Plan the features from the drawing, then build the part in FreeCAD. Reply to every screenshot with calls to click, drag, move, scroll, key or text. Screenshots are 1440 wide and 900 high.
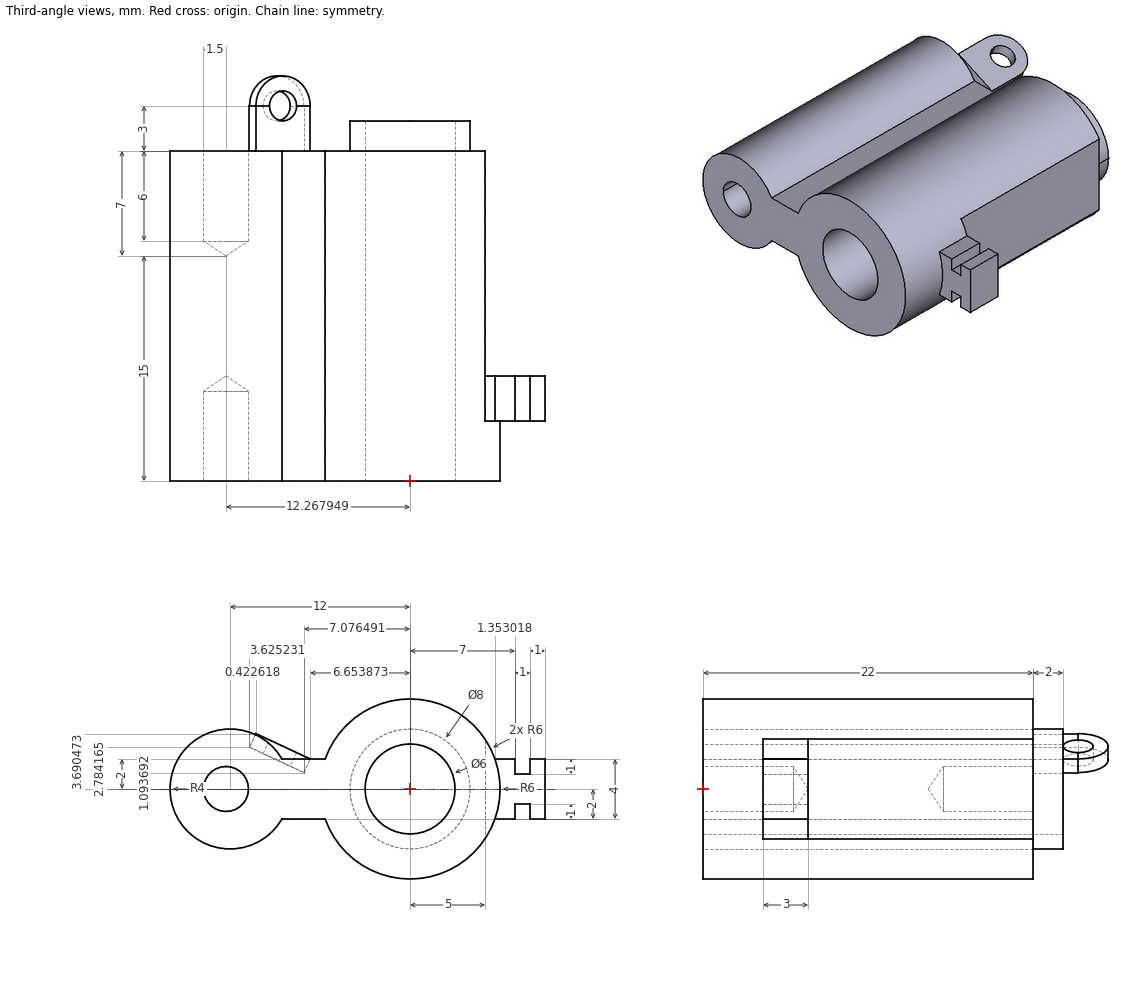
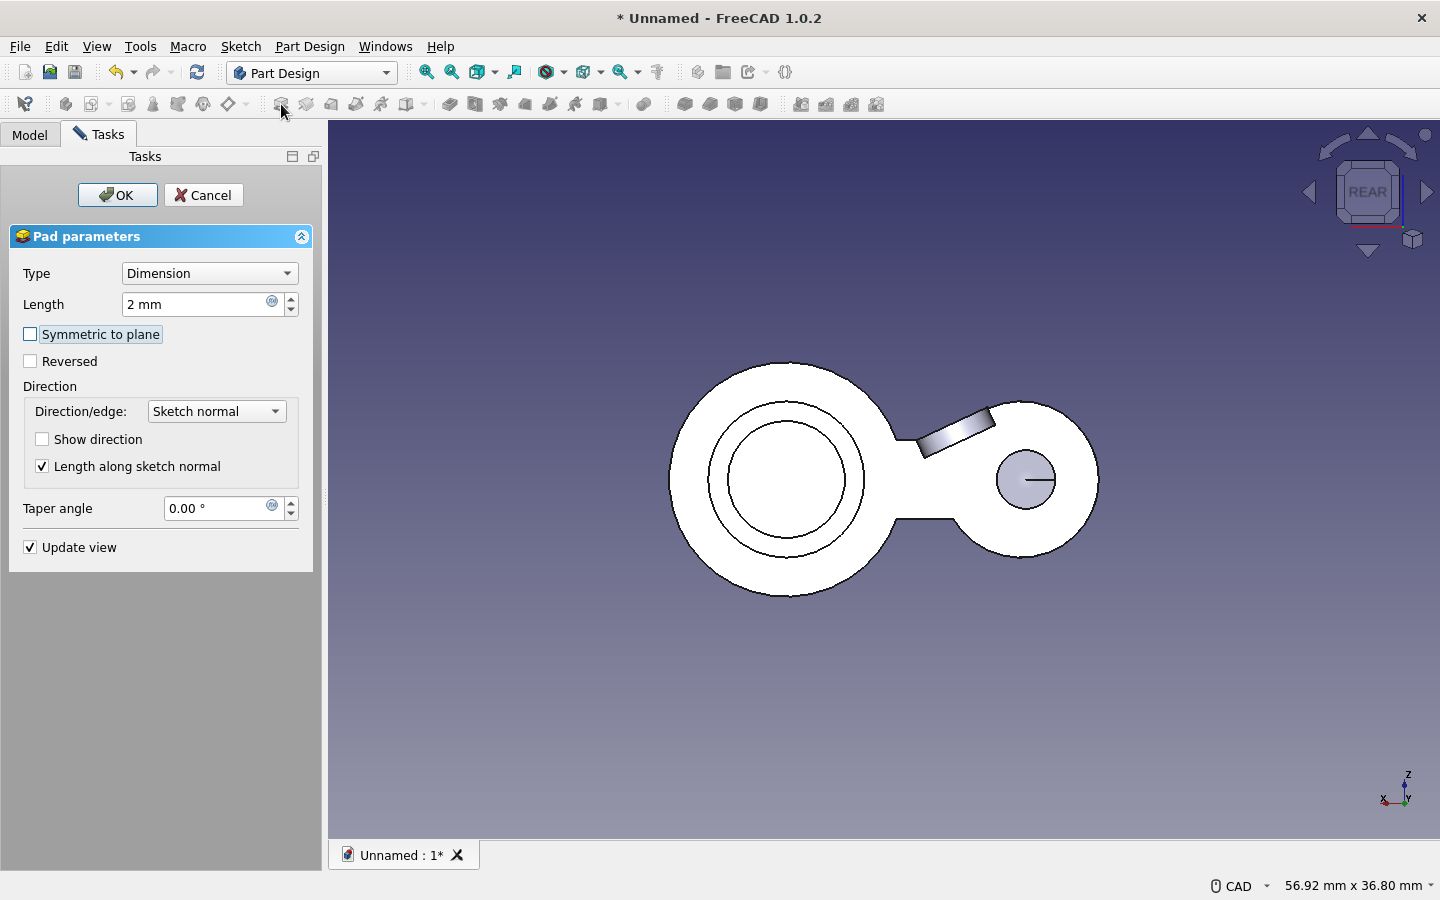
click(118, 195)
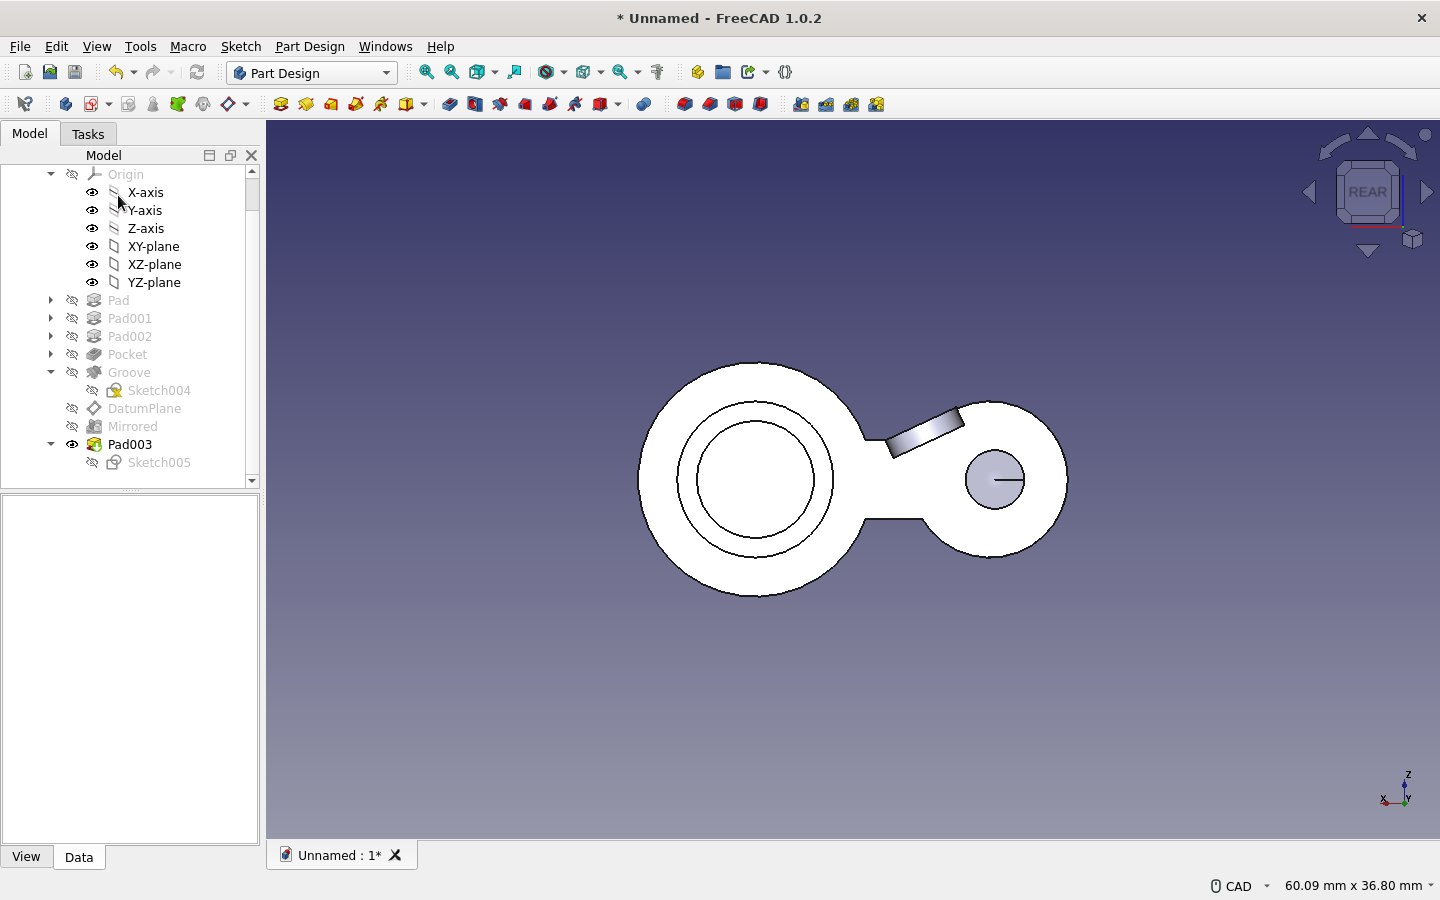
click(427, 72)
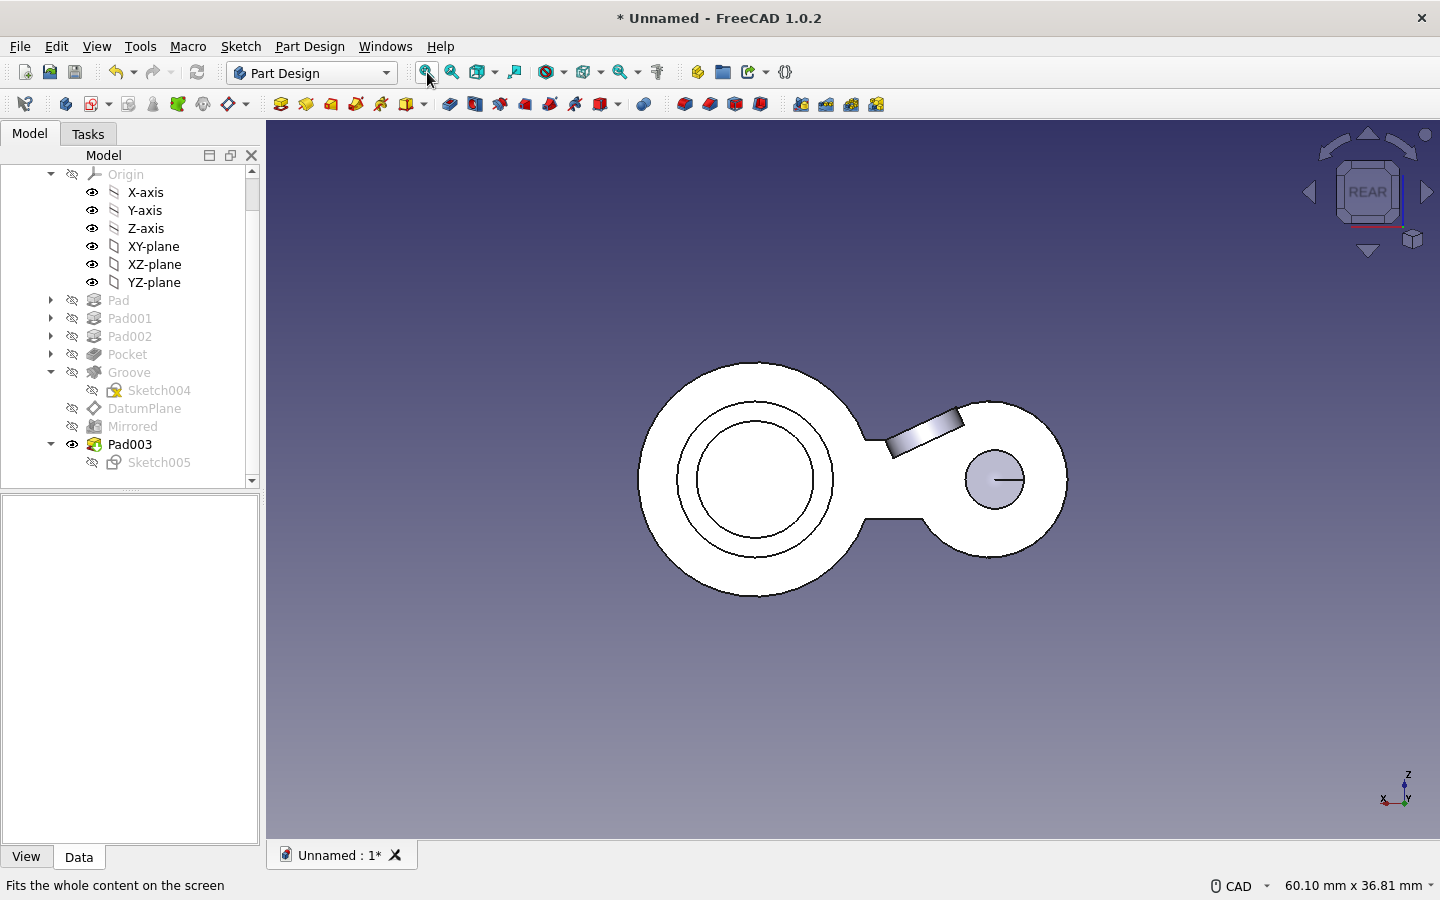
click(914, 478)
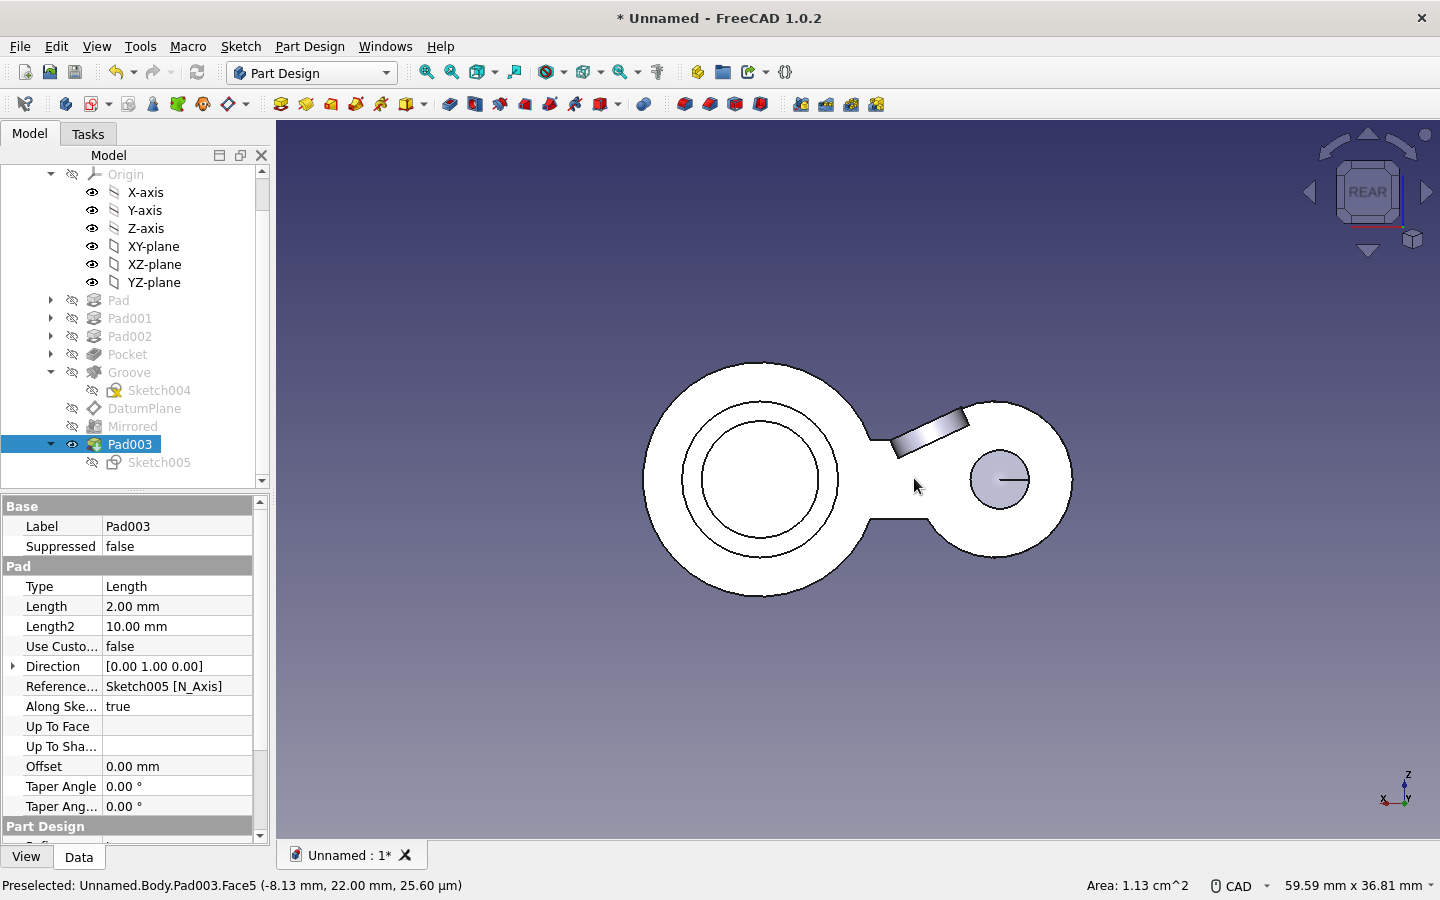
click(90, 104)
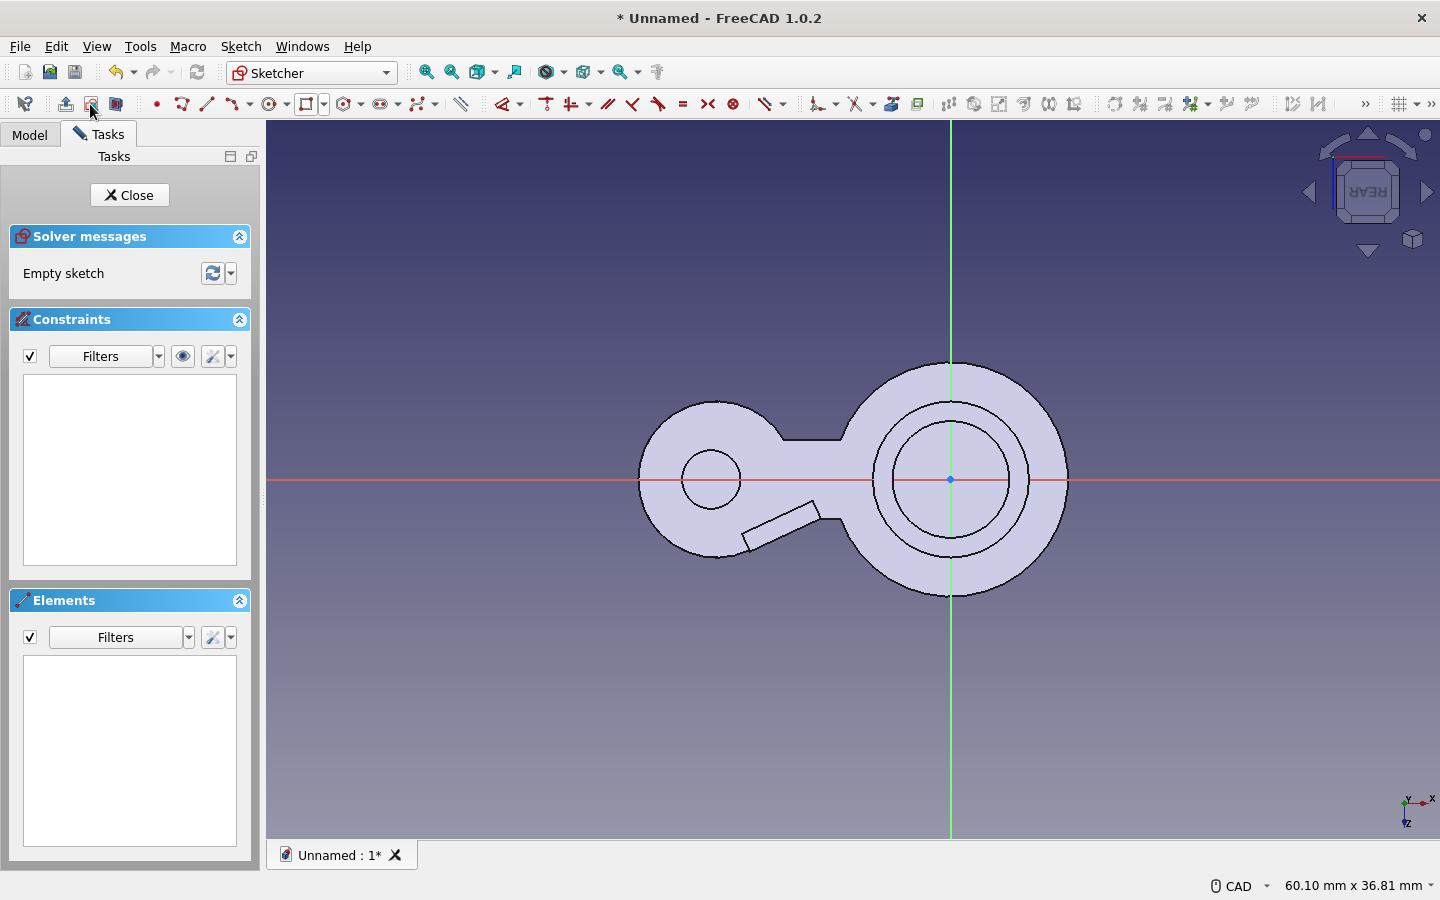
click(116, 104)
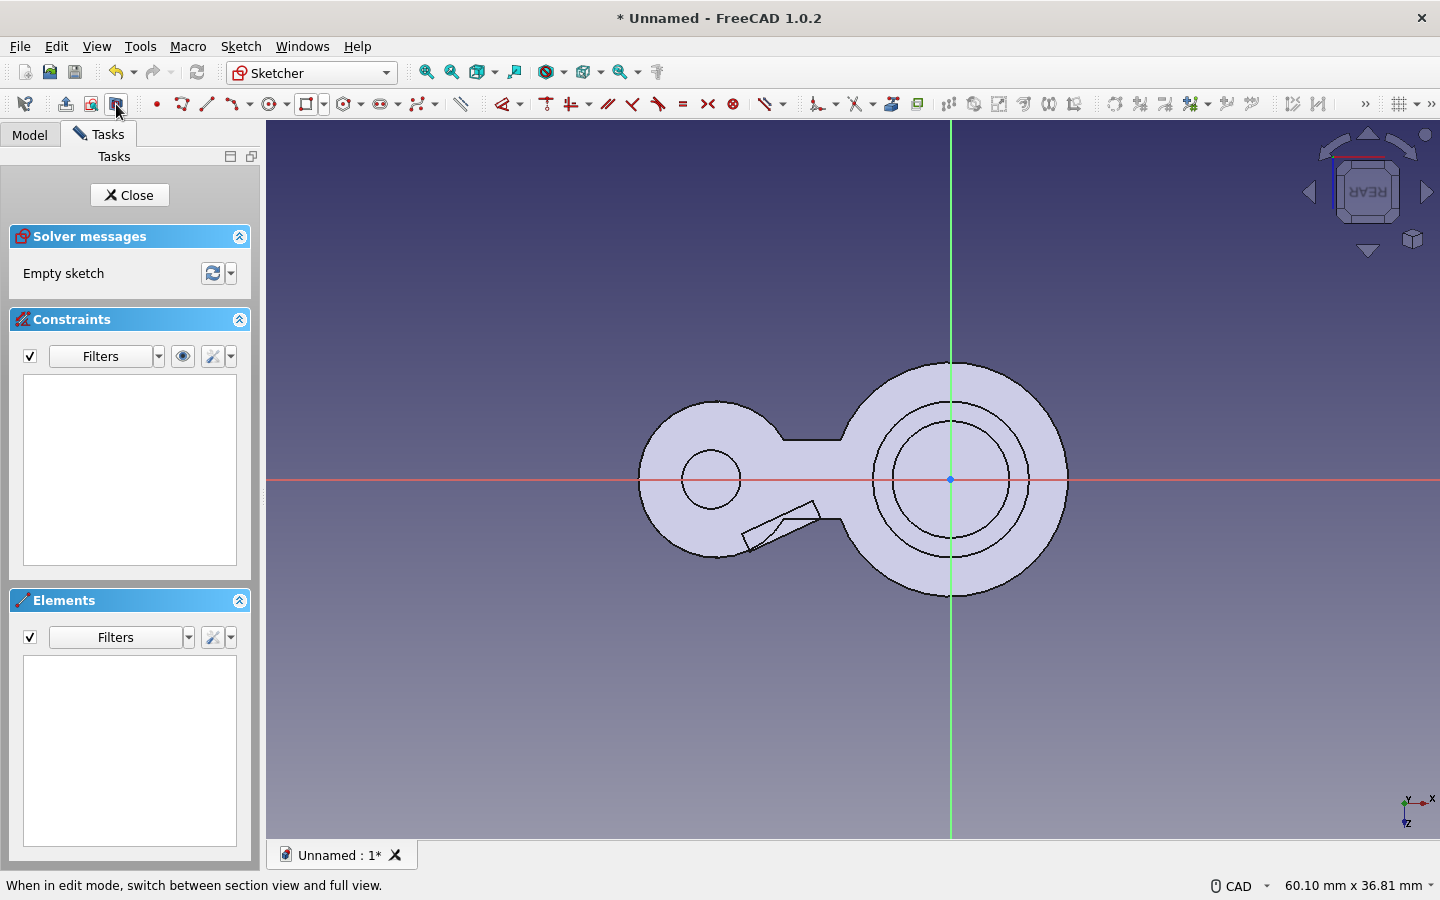
scroll(1005, 479, up, 7)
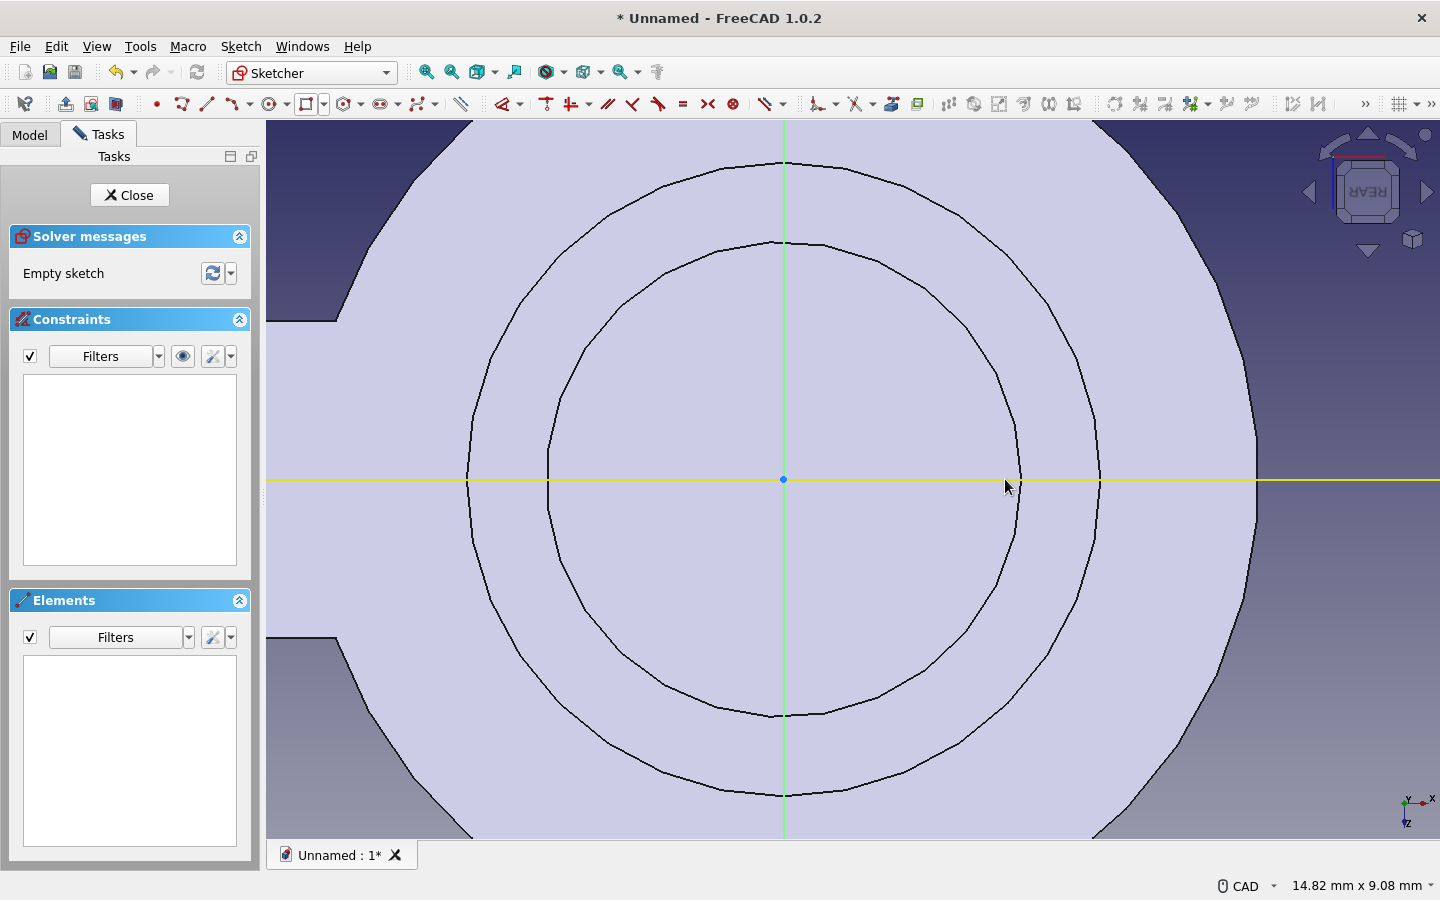
click(268, 104)